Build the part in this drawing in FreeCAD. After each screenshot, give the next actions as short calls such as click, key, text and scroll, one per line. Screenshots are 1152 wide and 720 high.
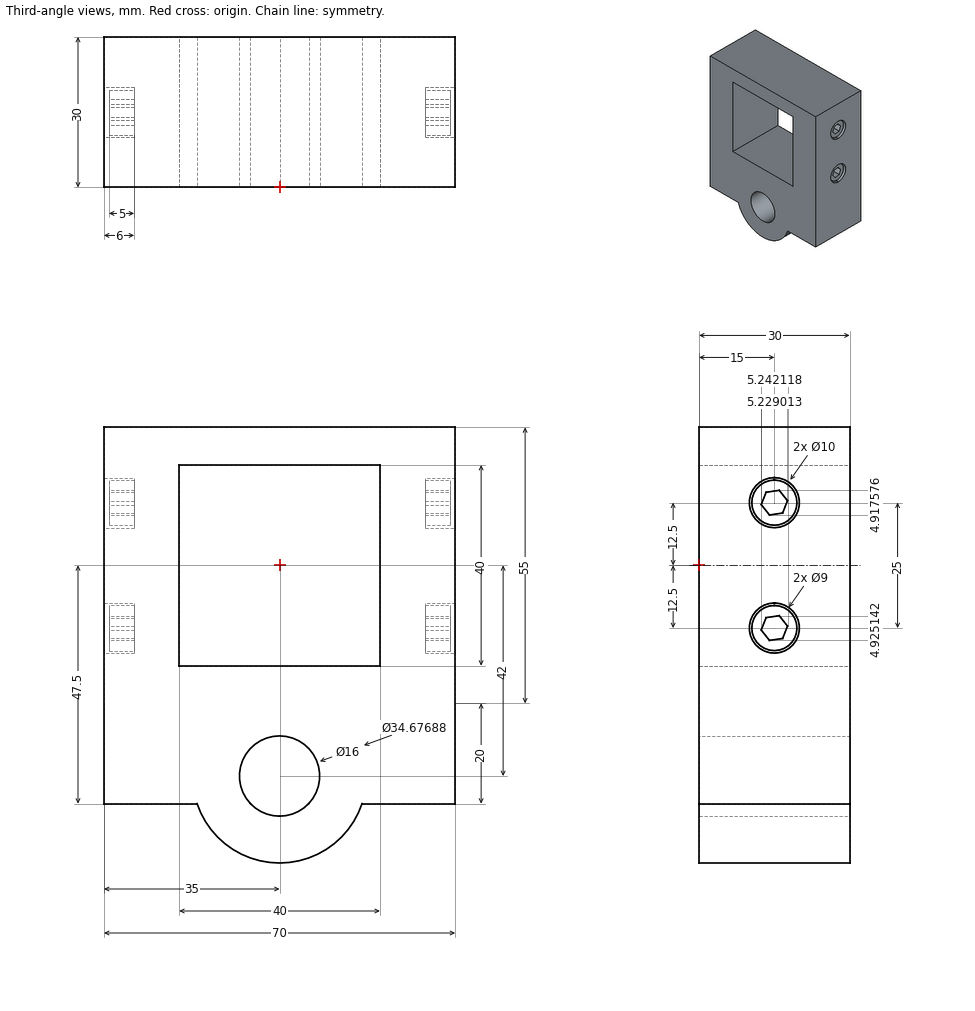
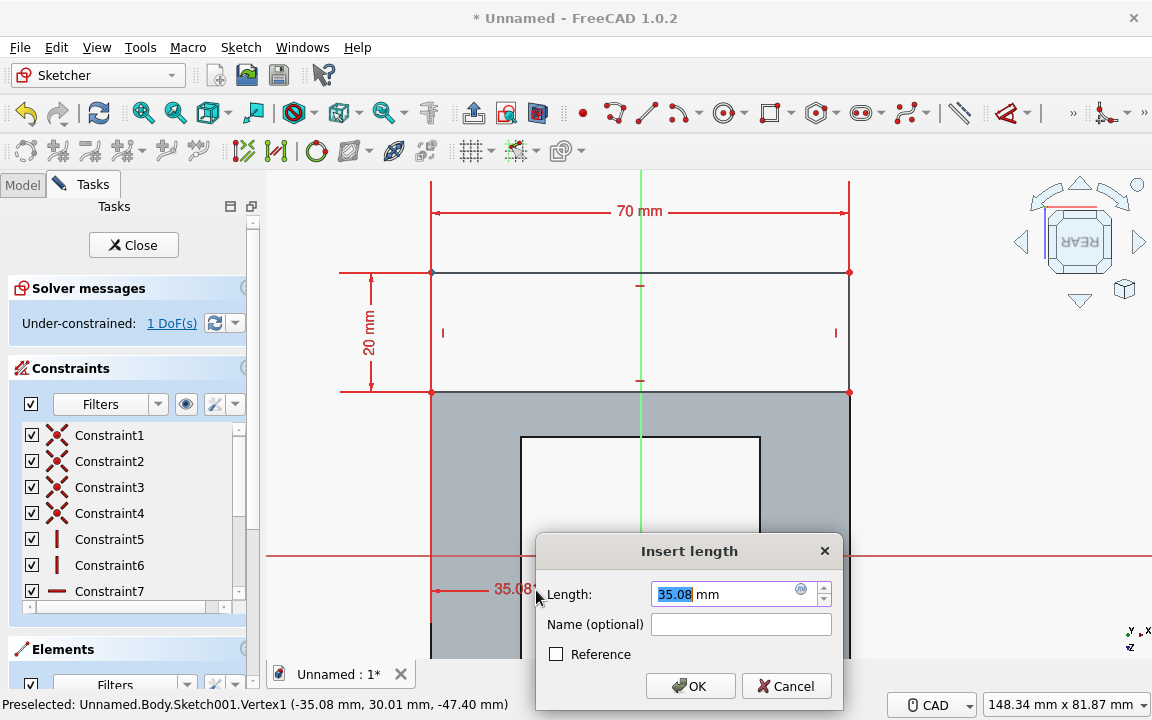
text(35)
key(Return)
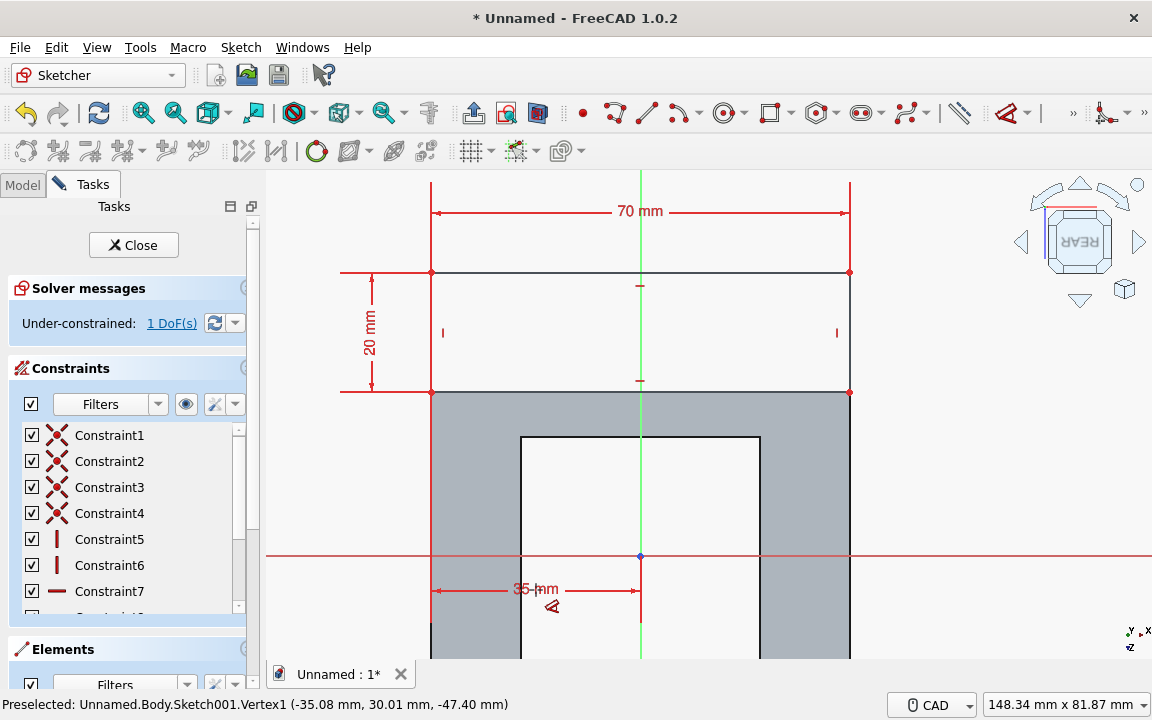
click(431, 273)
click(397, 415)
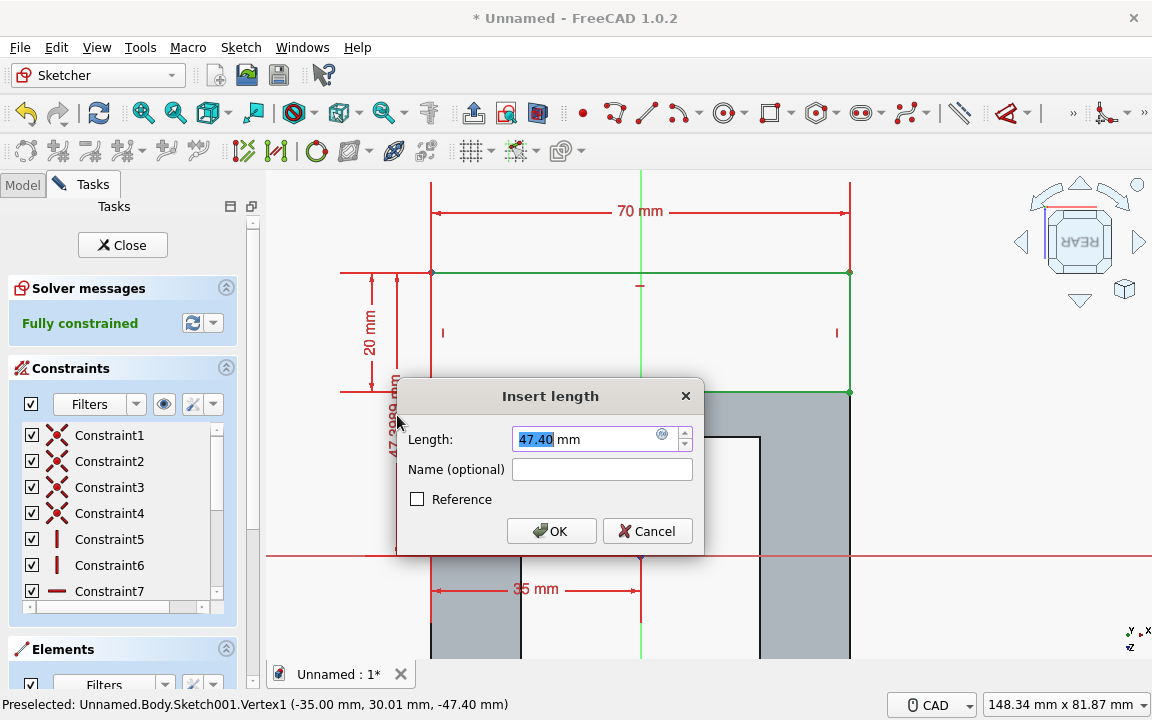
text(47.5)
key(Return)
key(Escape)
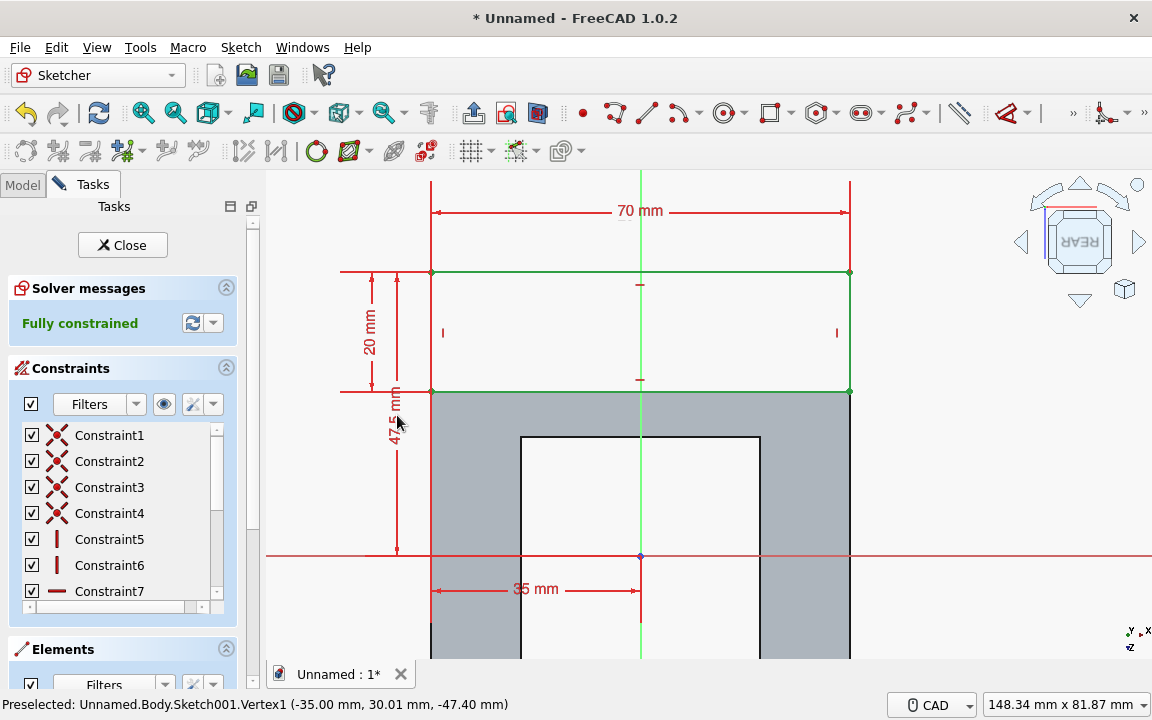
click(123, 245)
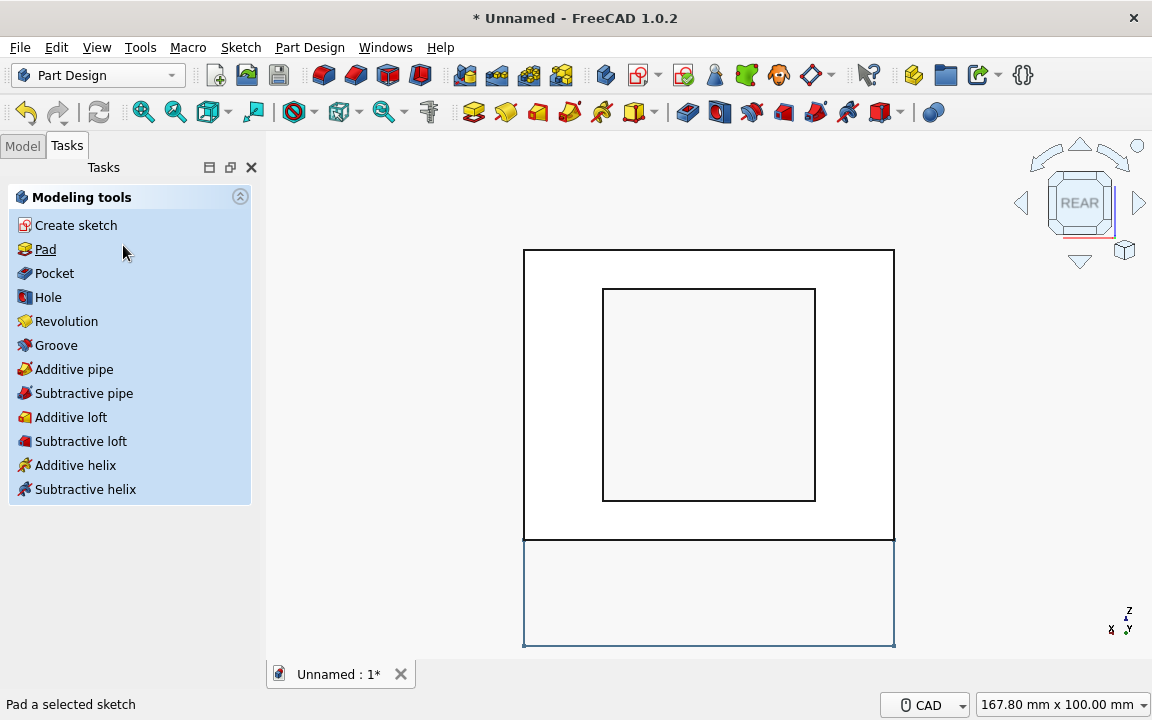
click(474, 112)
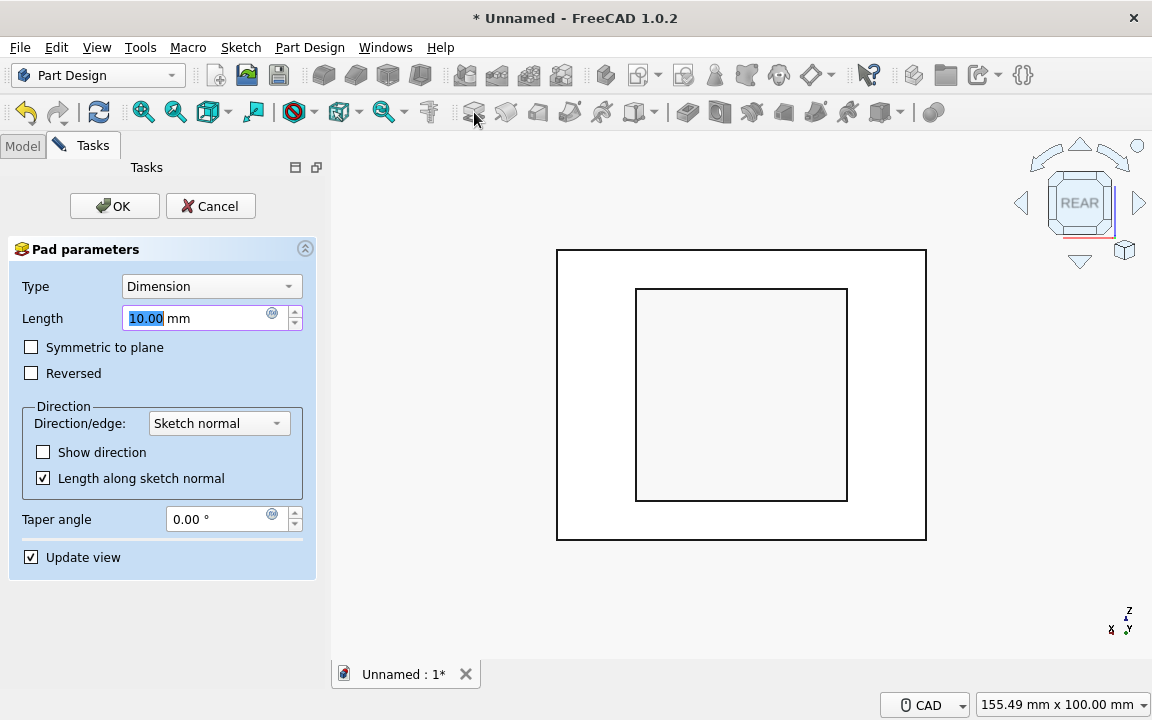
text(30)
key(Tab)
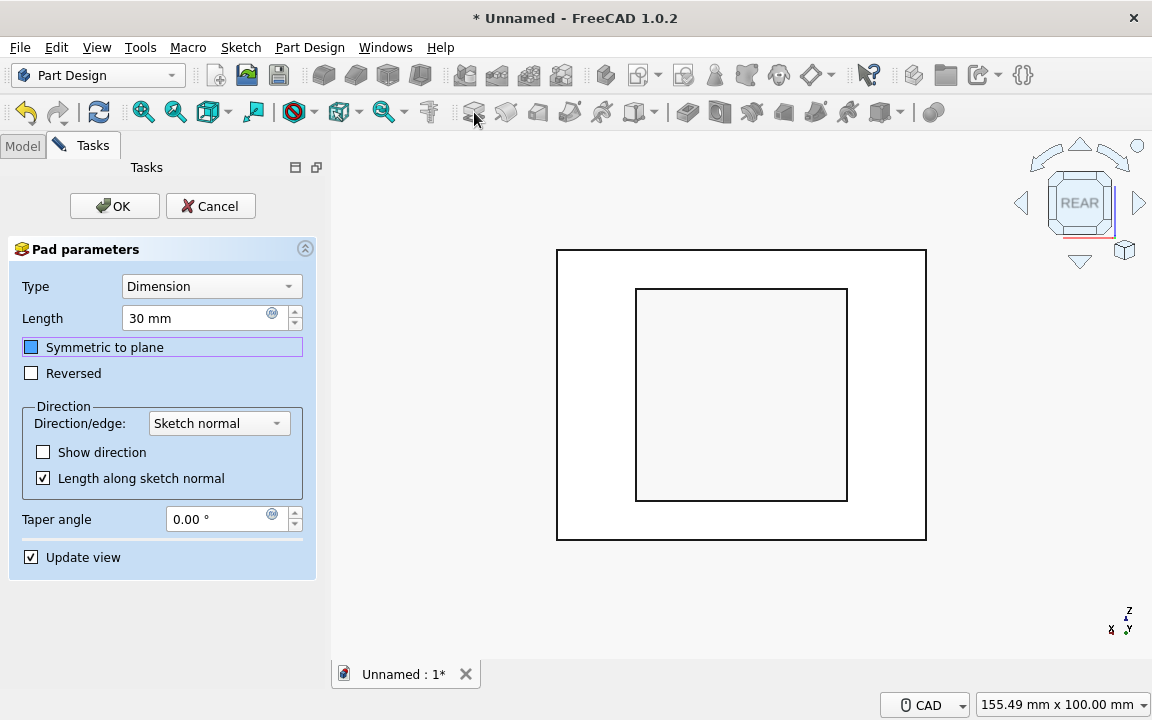
click(30, 373)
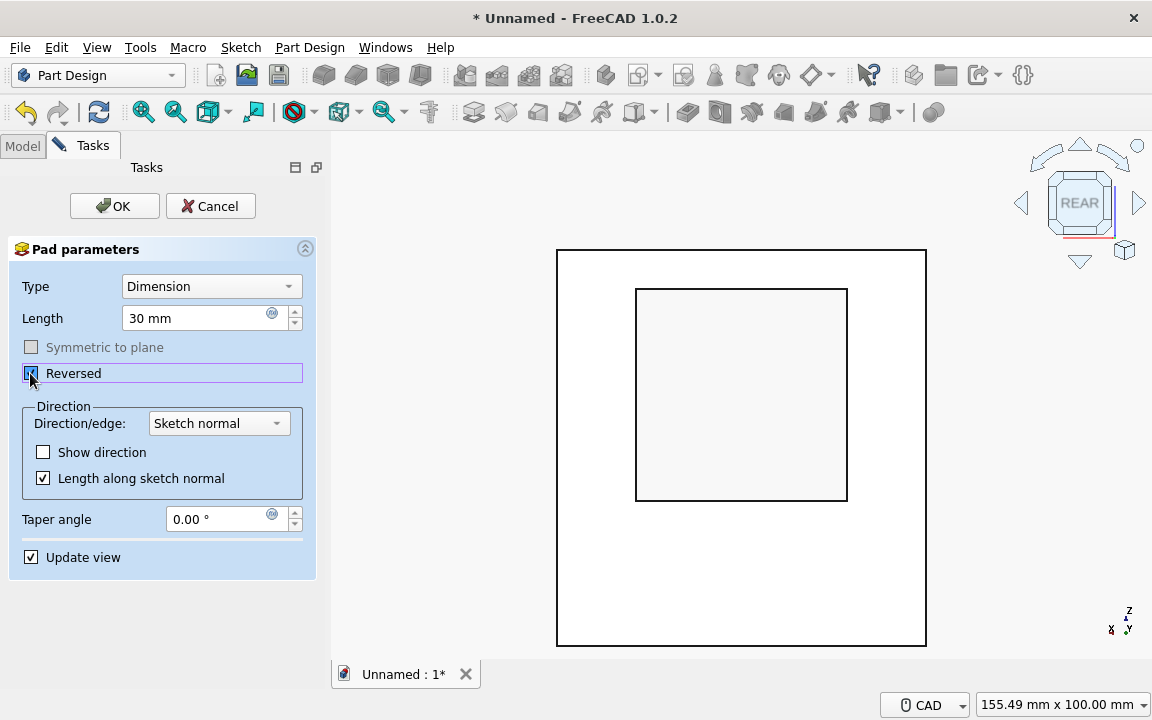
click(115, 206)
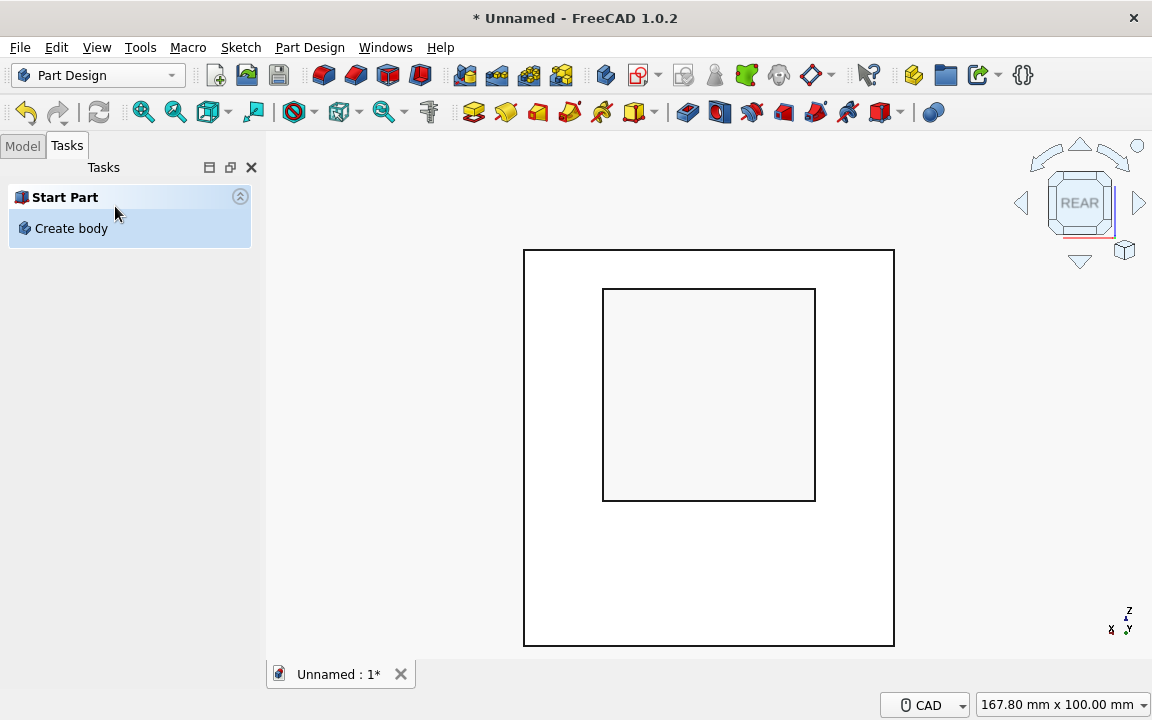
click(638, 76)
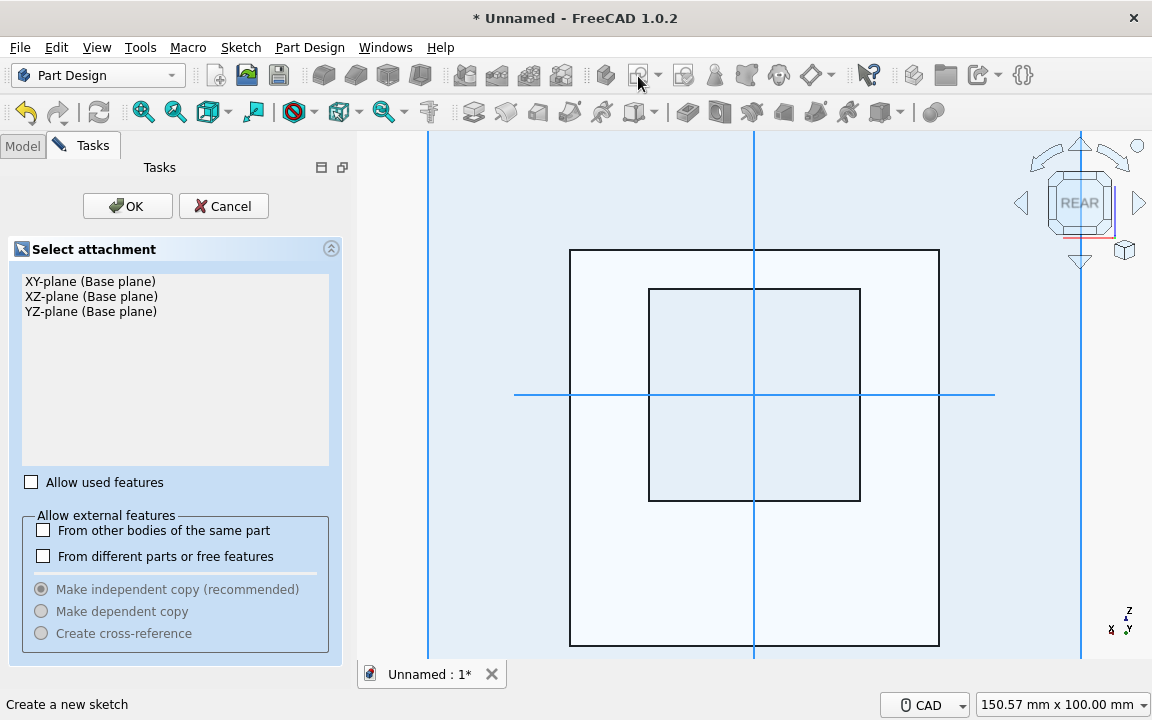
click(82, 296)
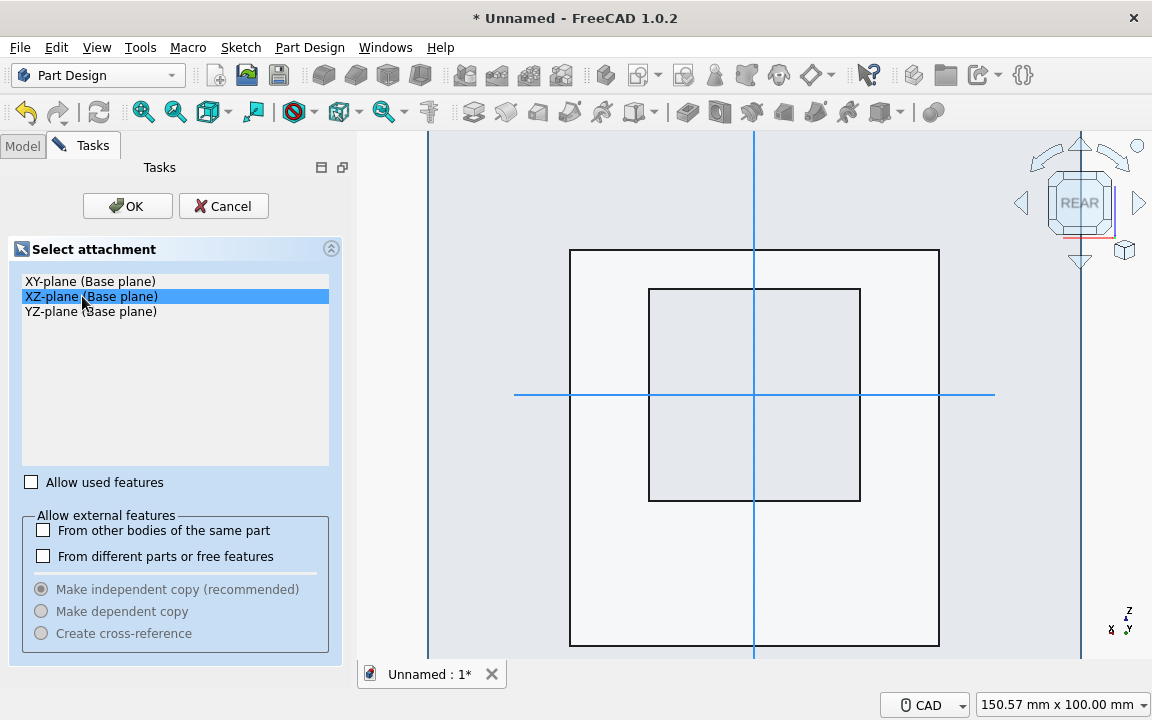
click(128, 206)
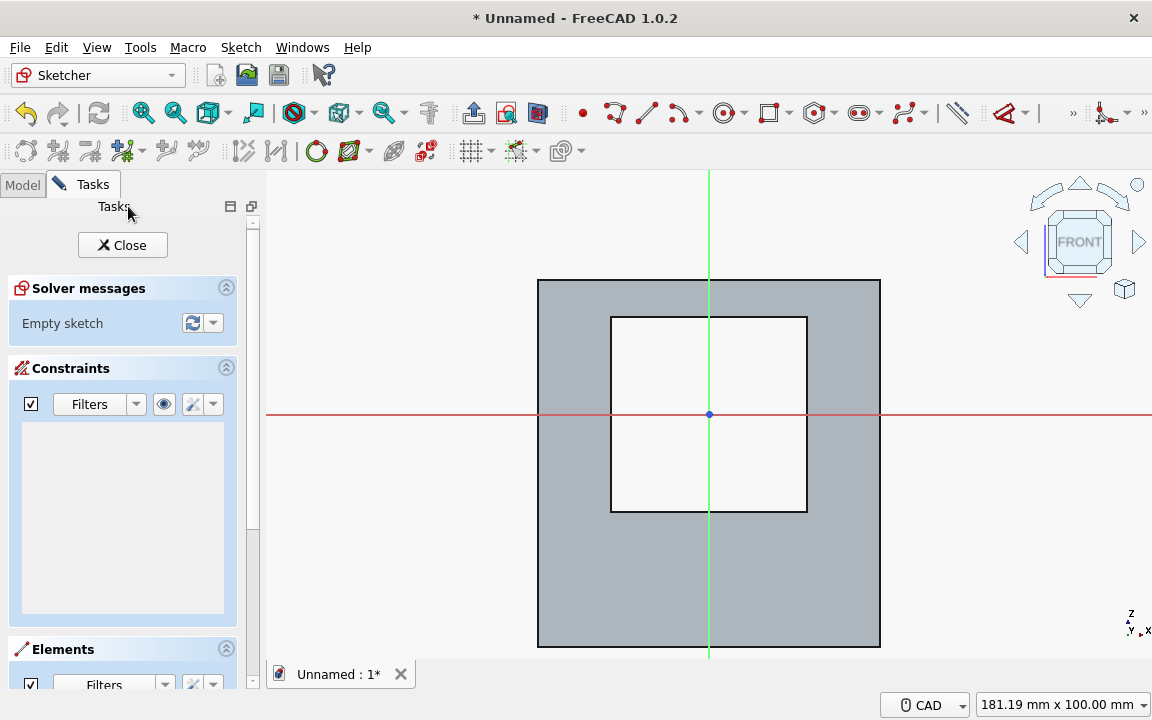
scroll(640, 414, down, 5)